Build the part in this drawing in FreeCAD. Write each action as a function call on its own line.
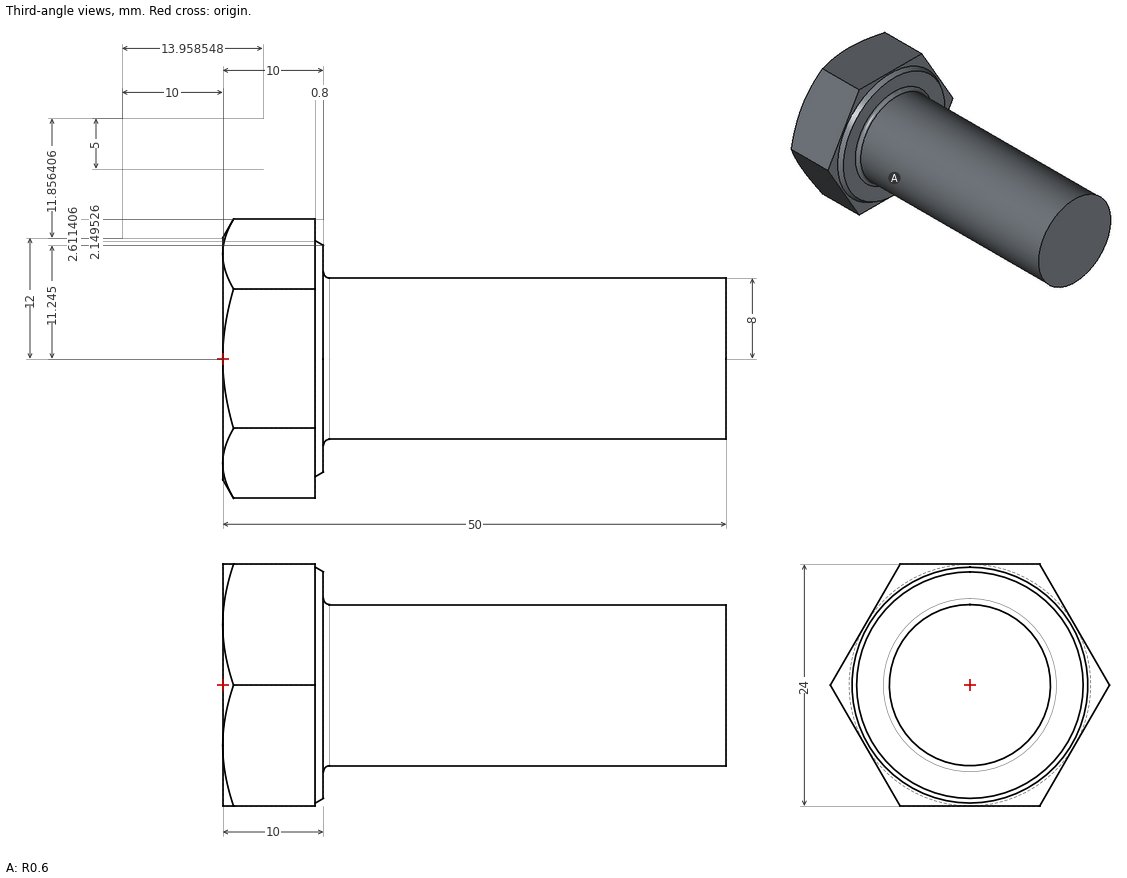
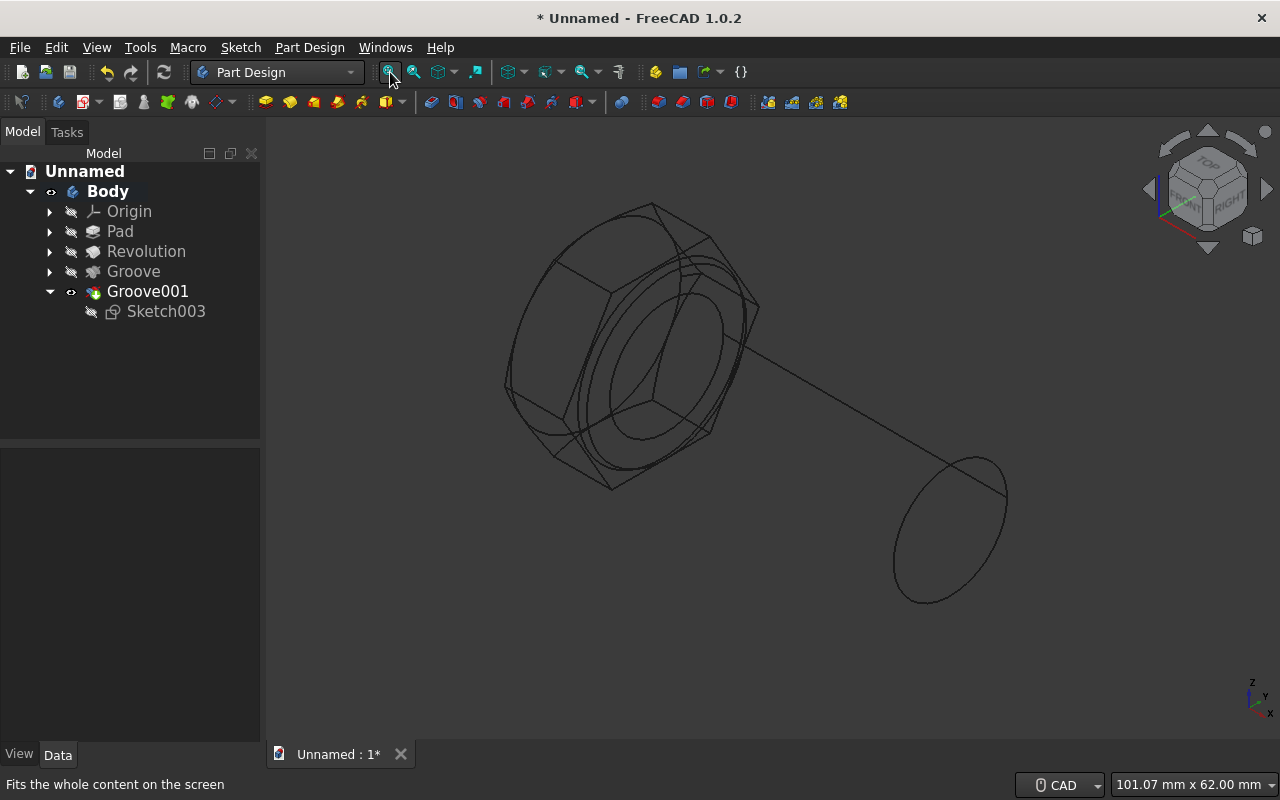
click(610, 398)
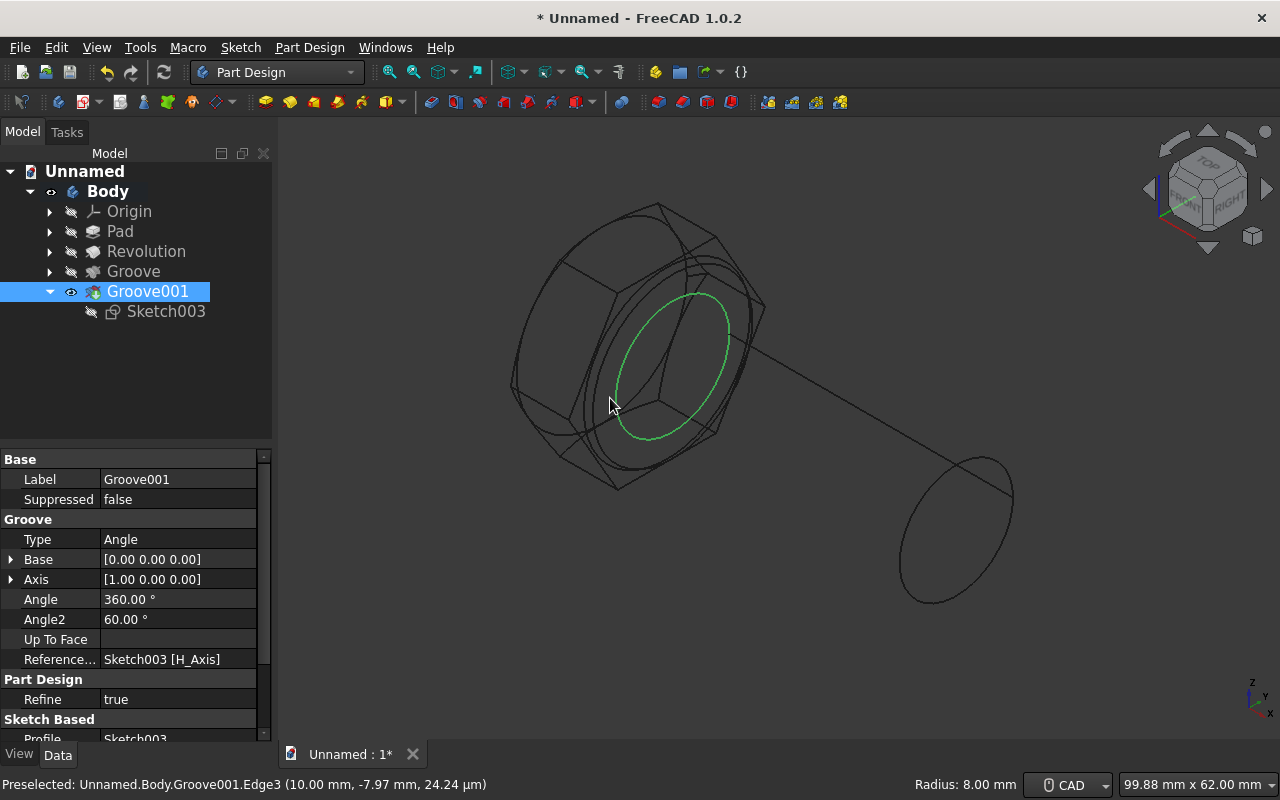
key(v)
key(1)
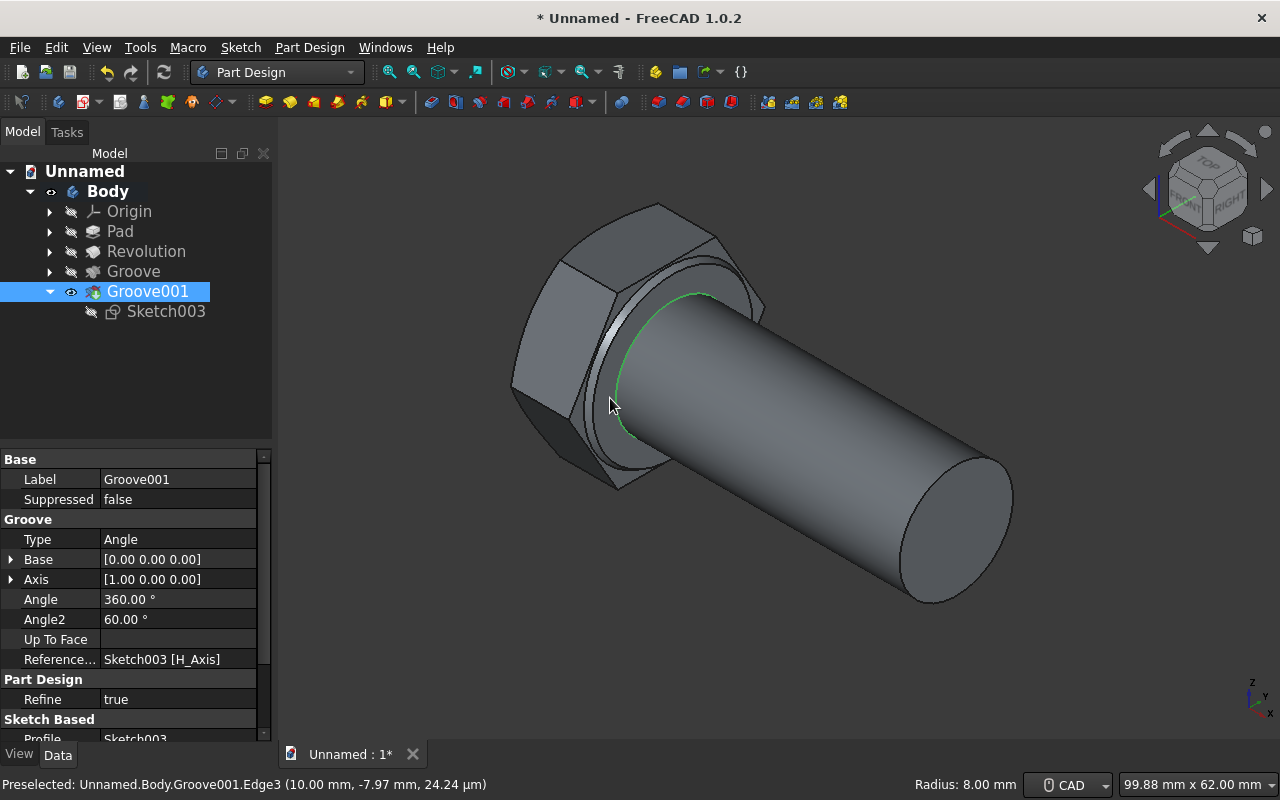
click(660, 102)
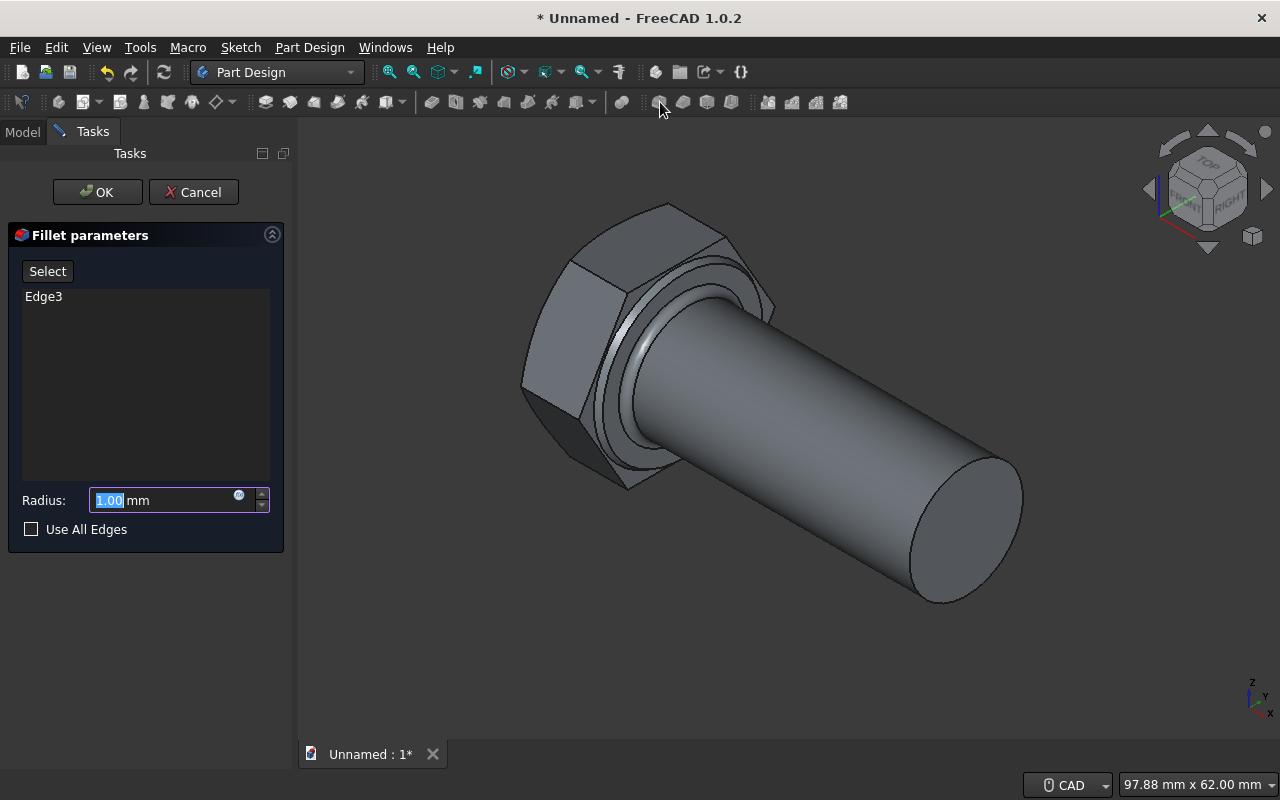
text(0.6)
key(Tab)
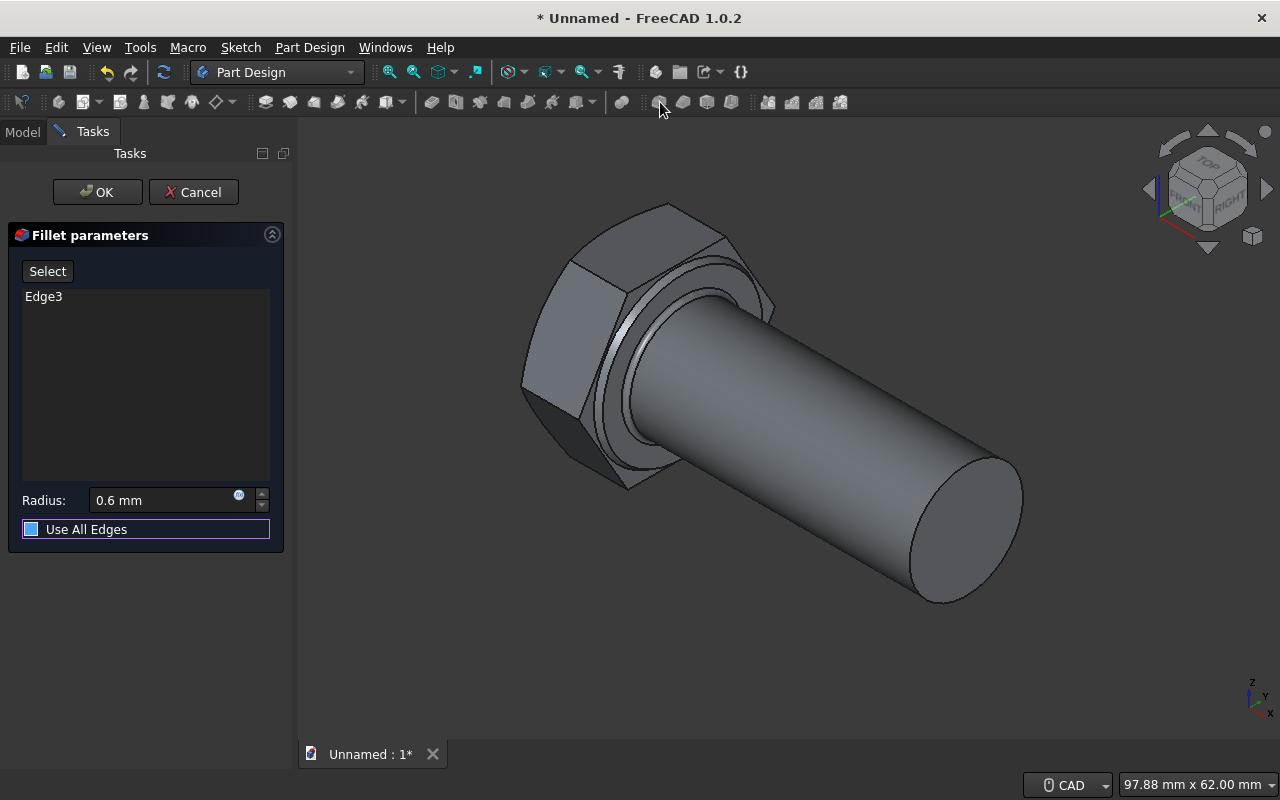
click(98, 192)